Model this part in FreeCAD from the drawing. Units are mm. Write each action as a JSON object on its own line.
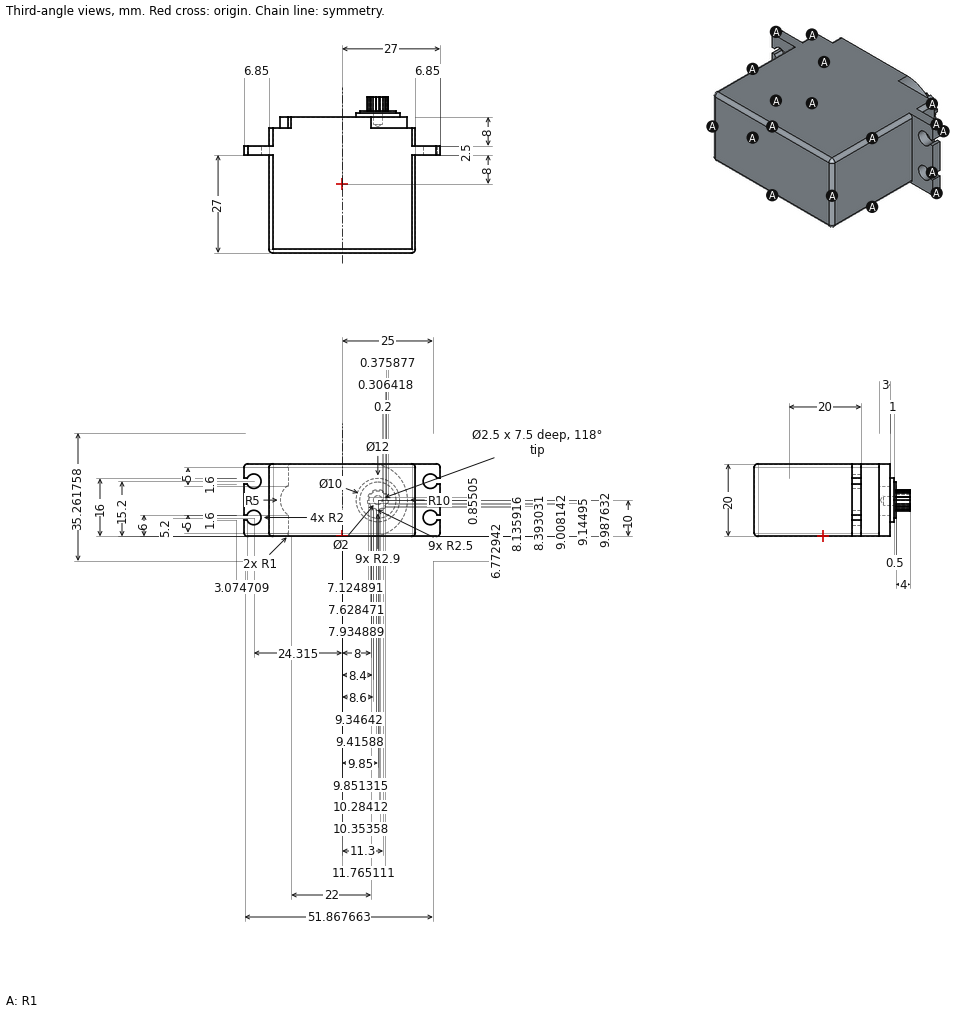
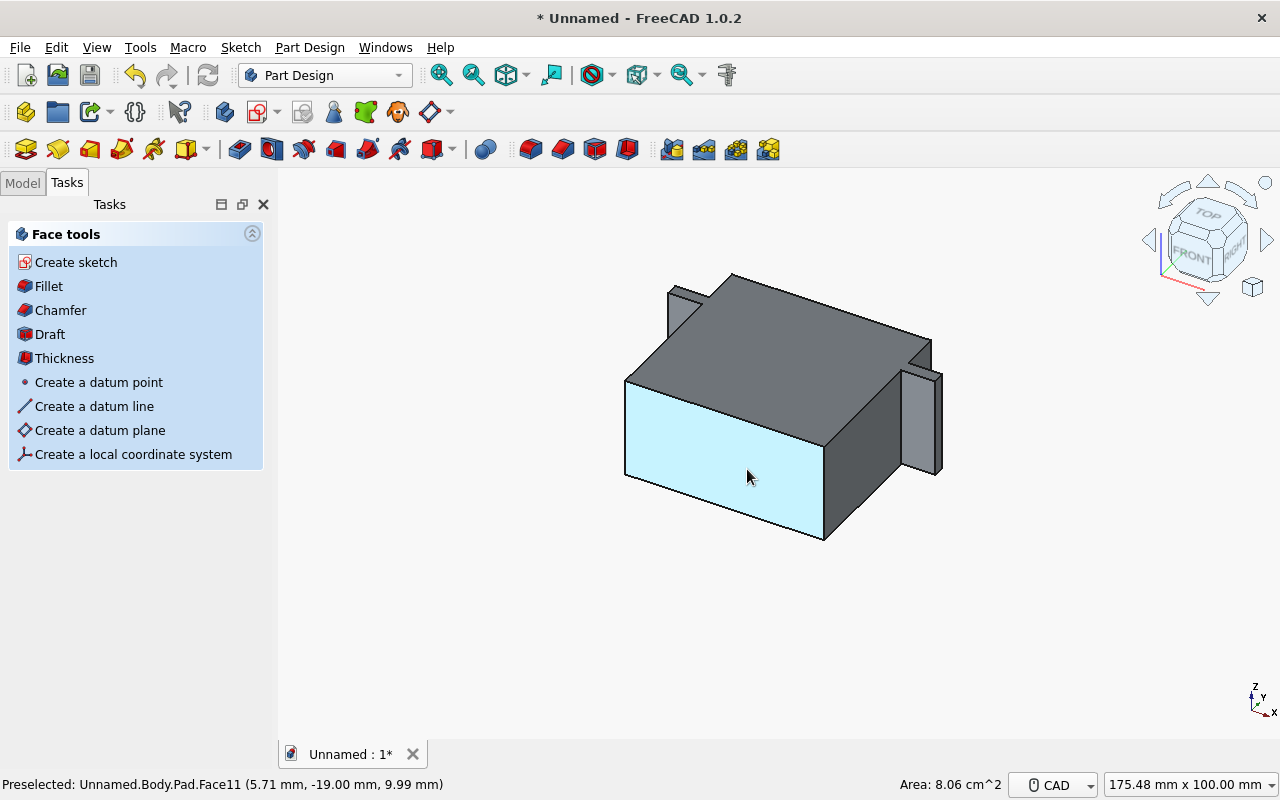
{"action": "left_click", "coordinate": [863, 408], "text": "ctrl"}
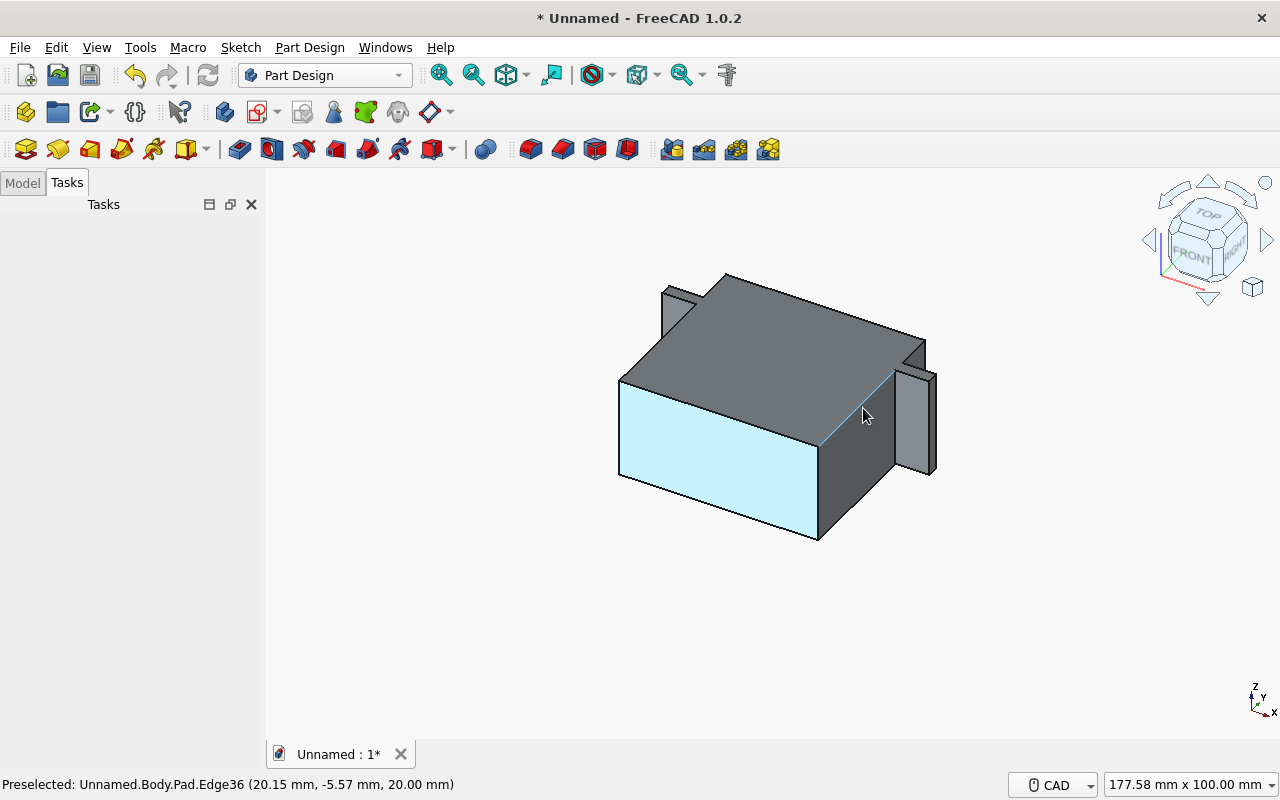
{"action": "left_click", "coordinate": [934, 376], "text": "ctrl"}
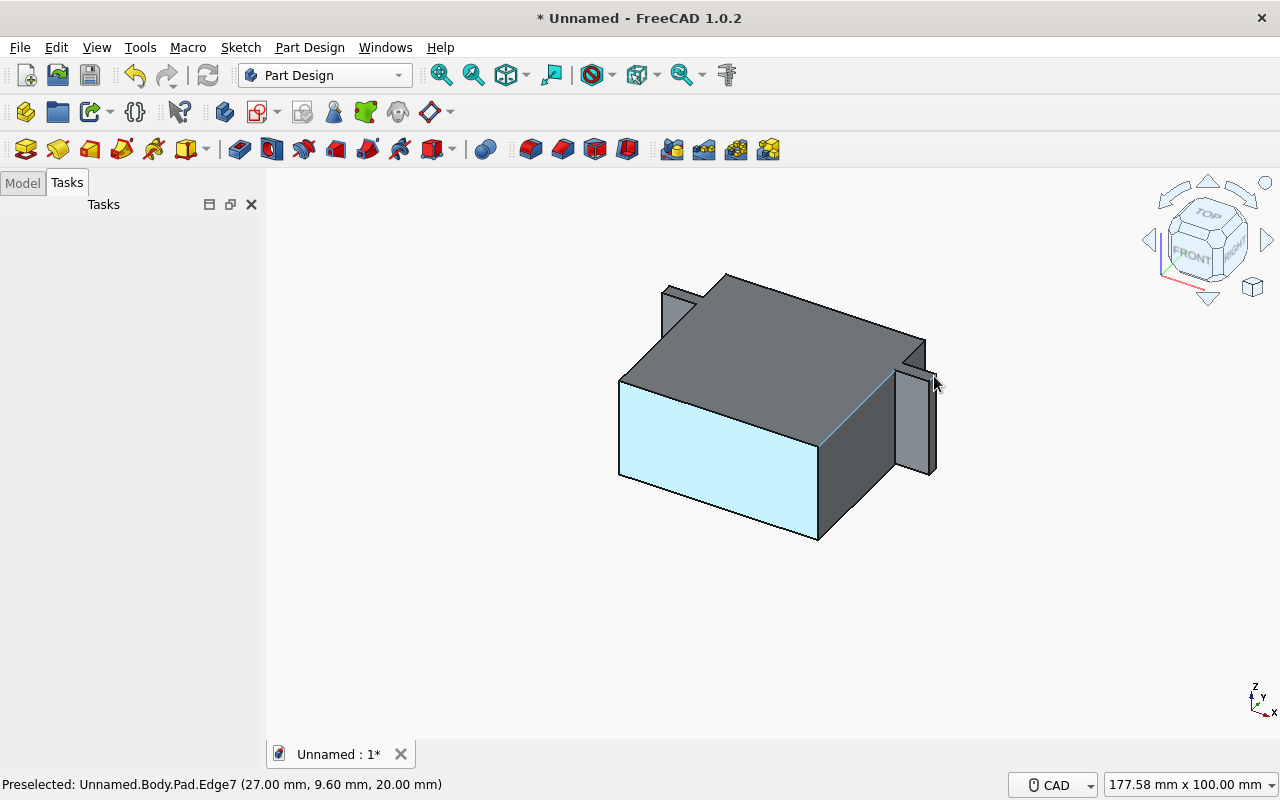
{"action": "left_click", "coordinate": [914, 351], "text": "ctrl"}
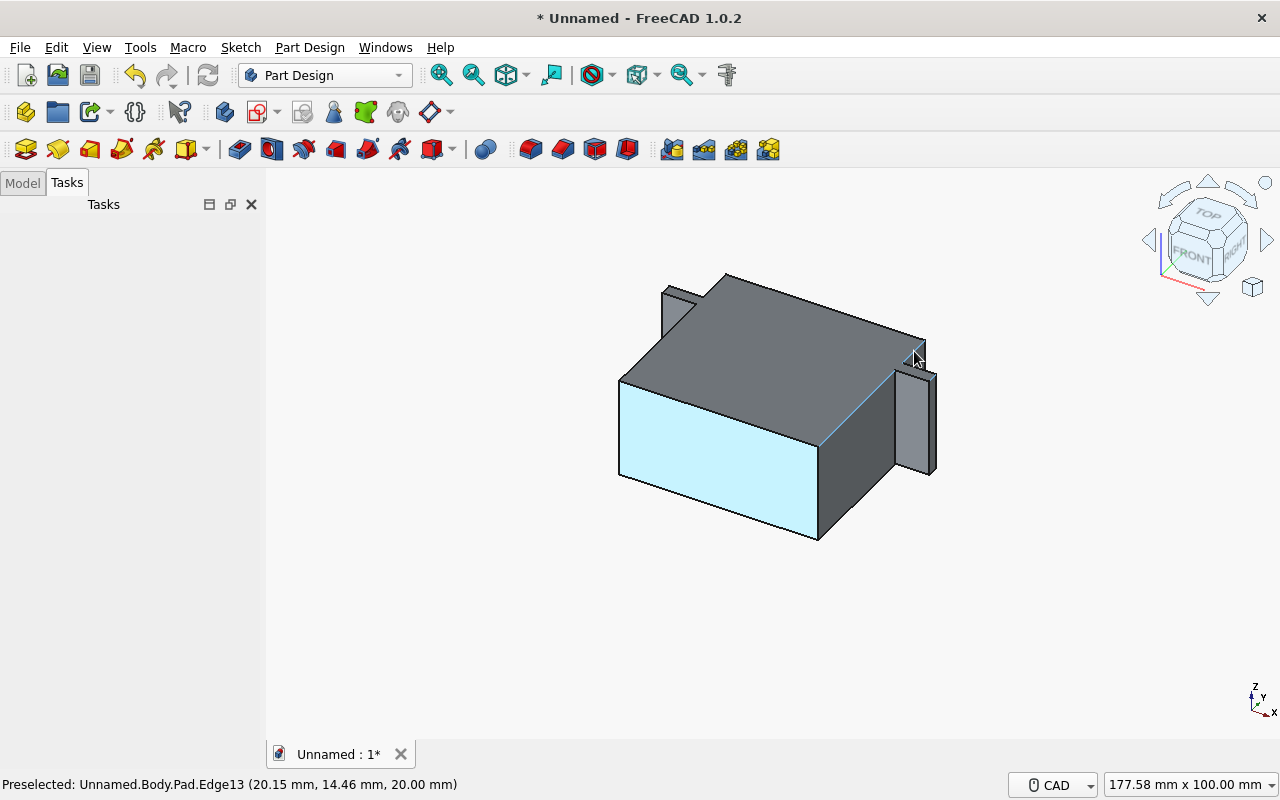
{"action": "scroll", "coordinate": [666, 289], "scroll_direction": "up", "scroll_amount": 6}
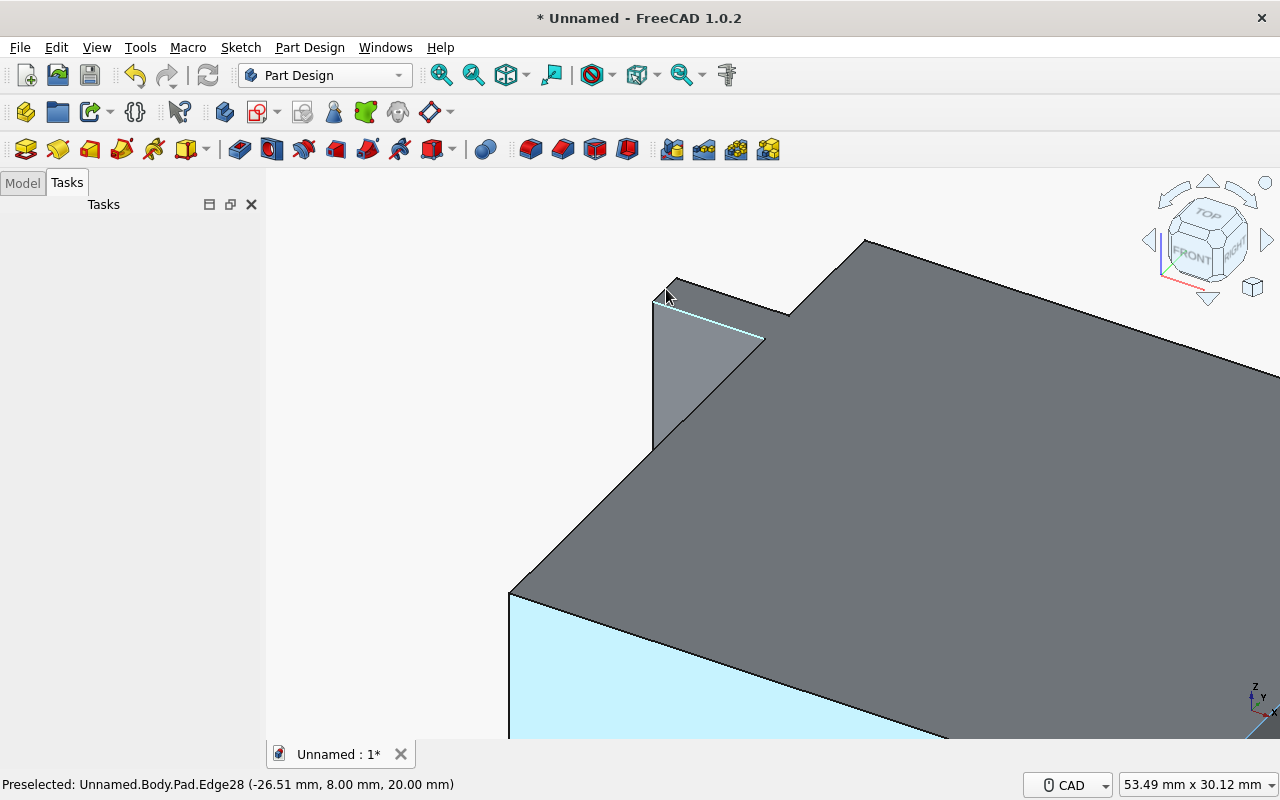
{"action": "left_click", "coordinate": [442, 76]}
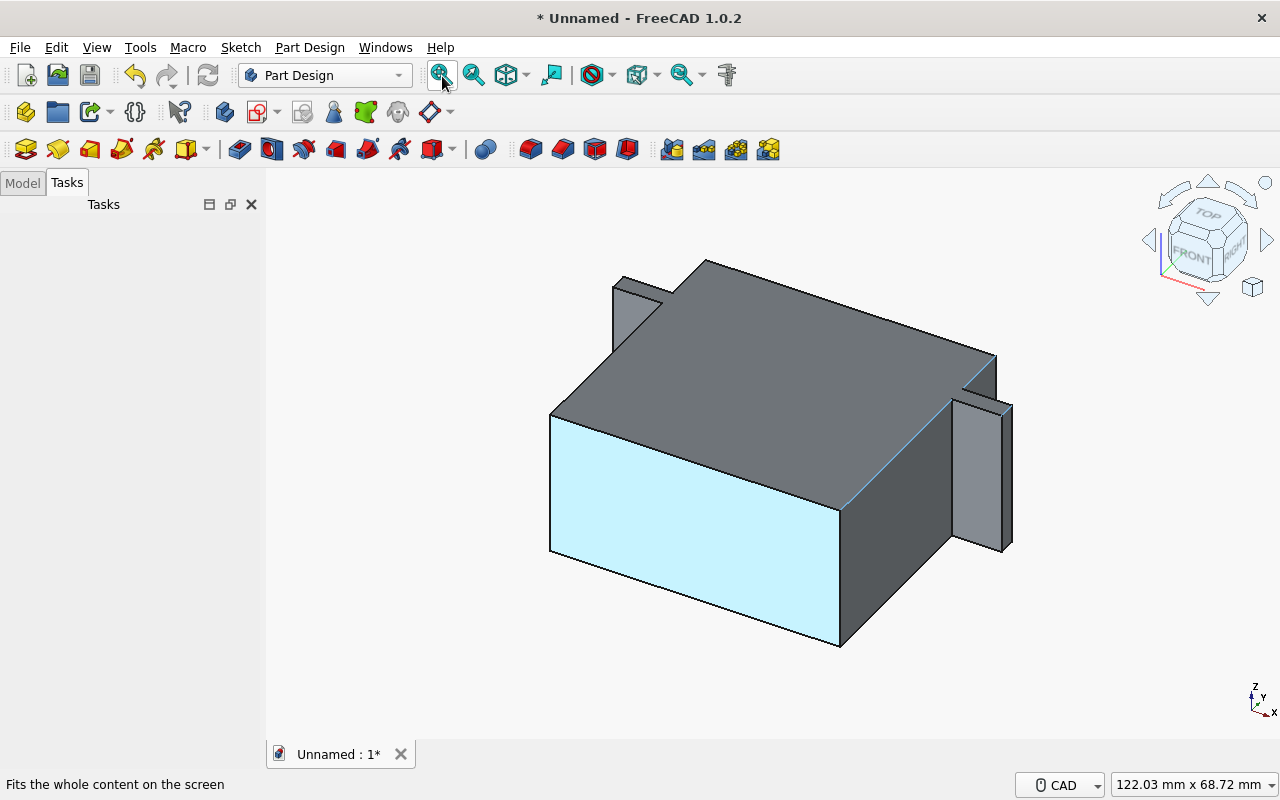
{"action": "key", "text": "0"}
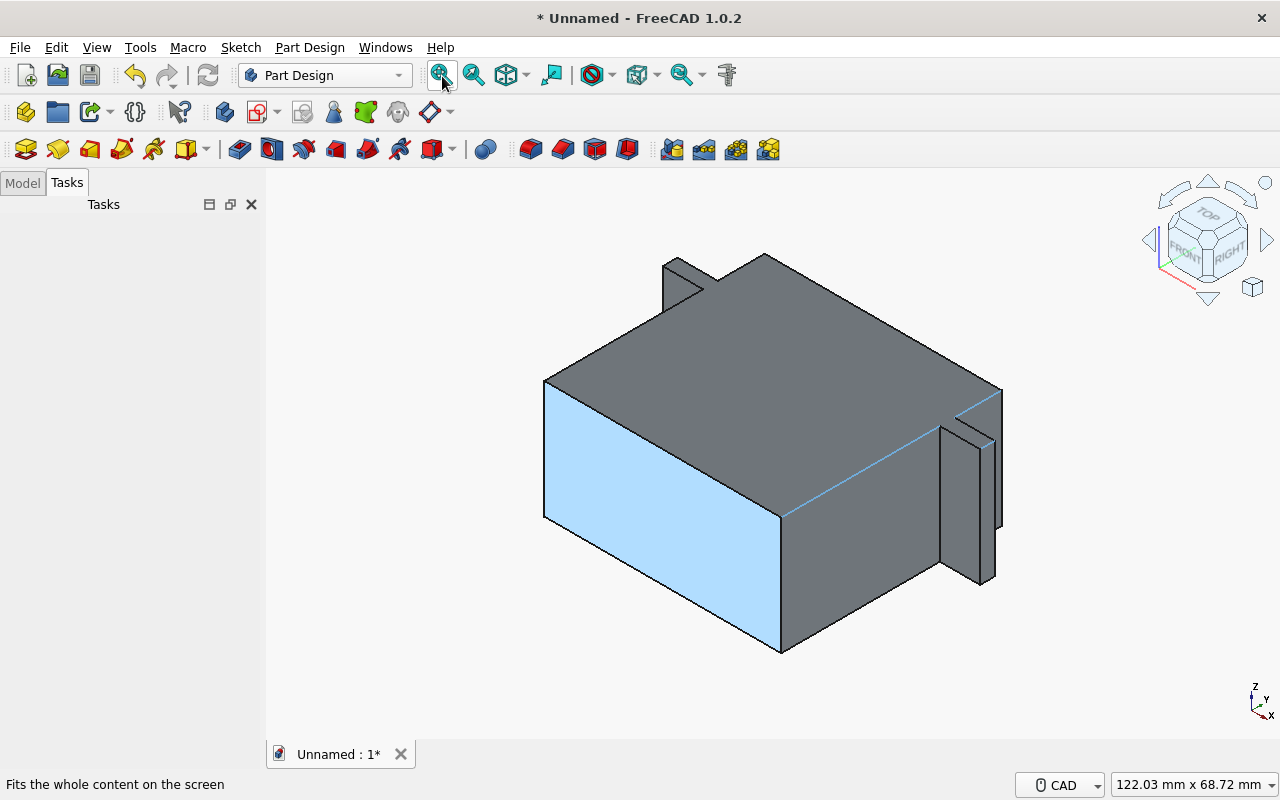
{"action": "scroll", "coordinate": [670, 261], "scroll_direction": "up", "scroll_amount": 4}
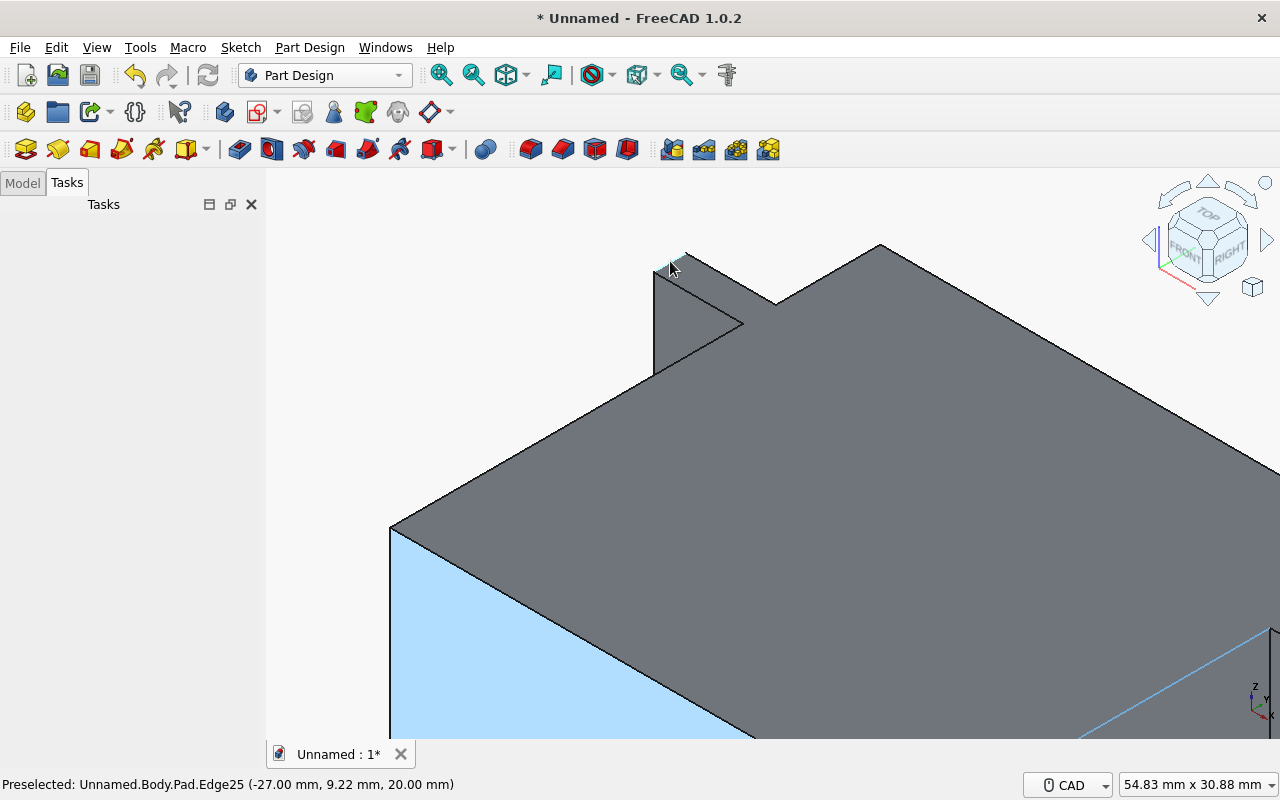
{"action": "left_click", "coordinate": [442, 76]}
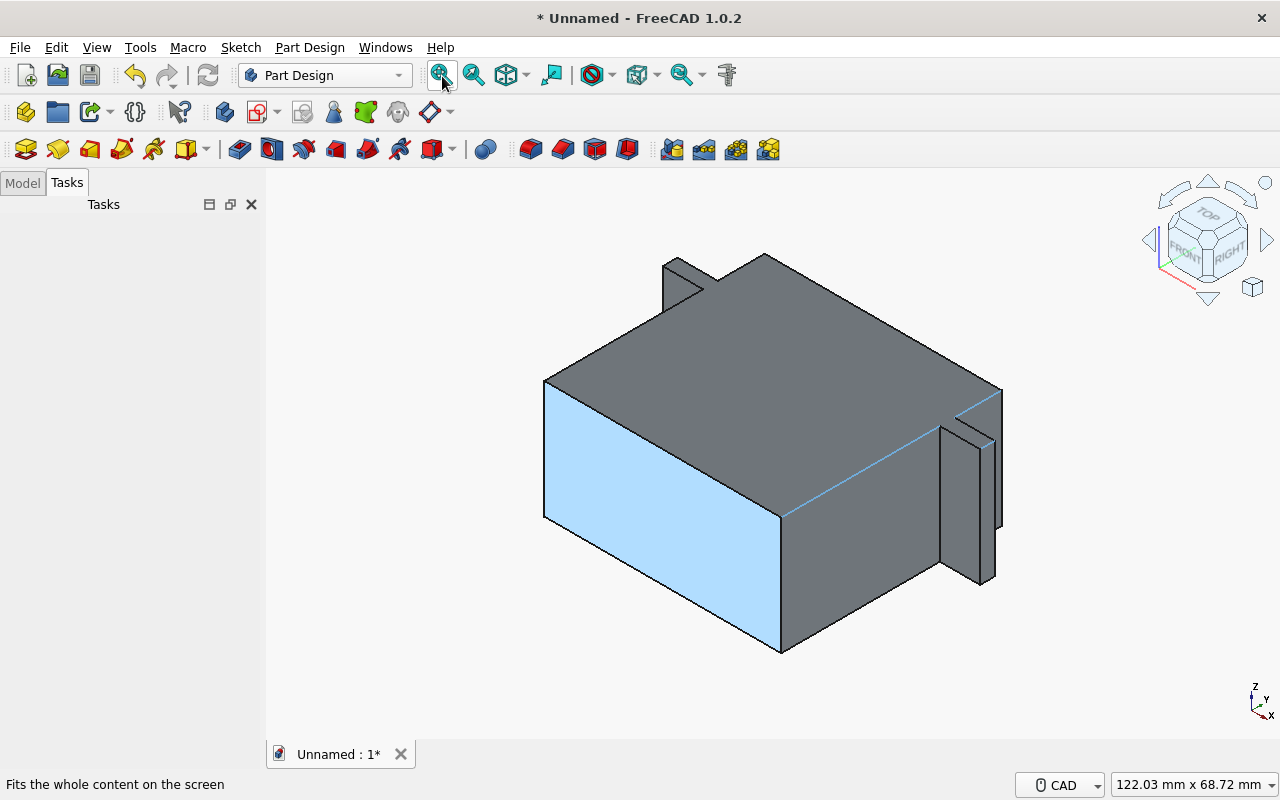
{"action": "key", "text": "2"}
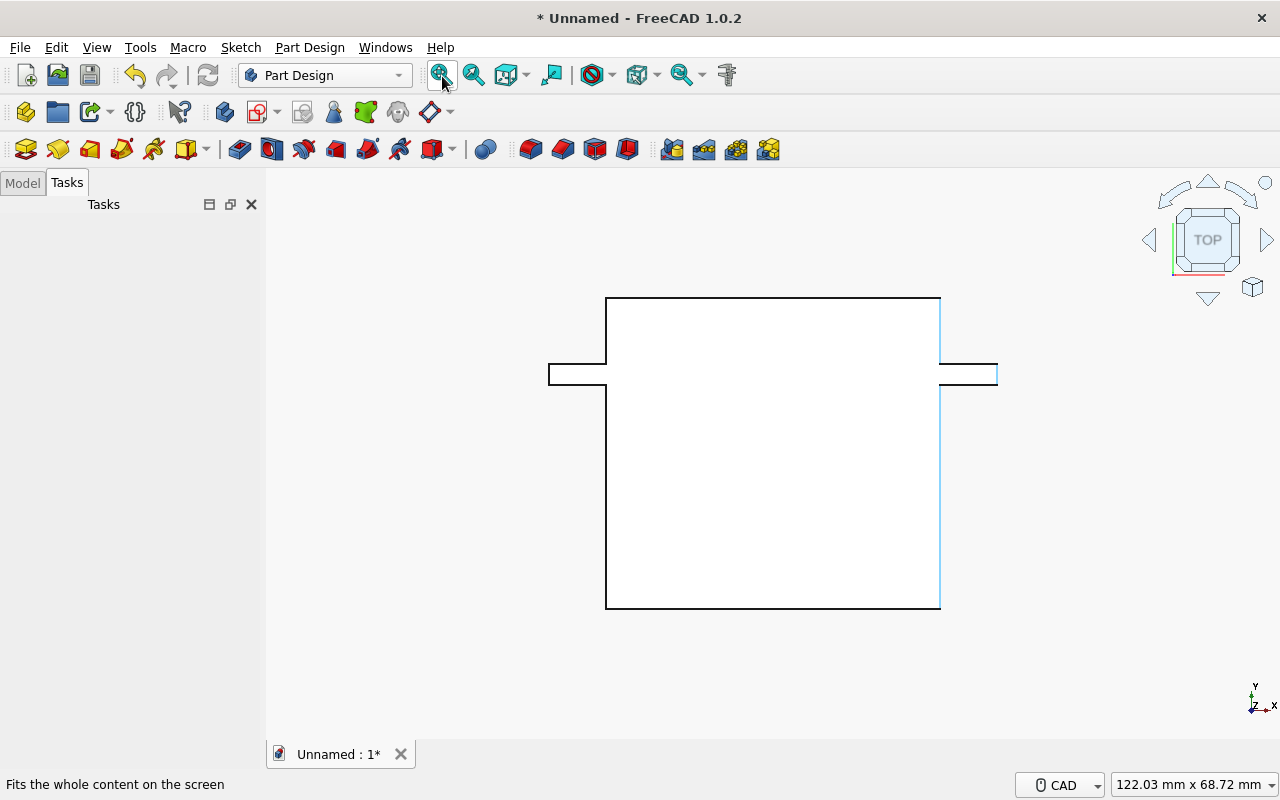
{"action": "left_click", "coordinate": [549, 374], "text": "ctrl"}